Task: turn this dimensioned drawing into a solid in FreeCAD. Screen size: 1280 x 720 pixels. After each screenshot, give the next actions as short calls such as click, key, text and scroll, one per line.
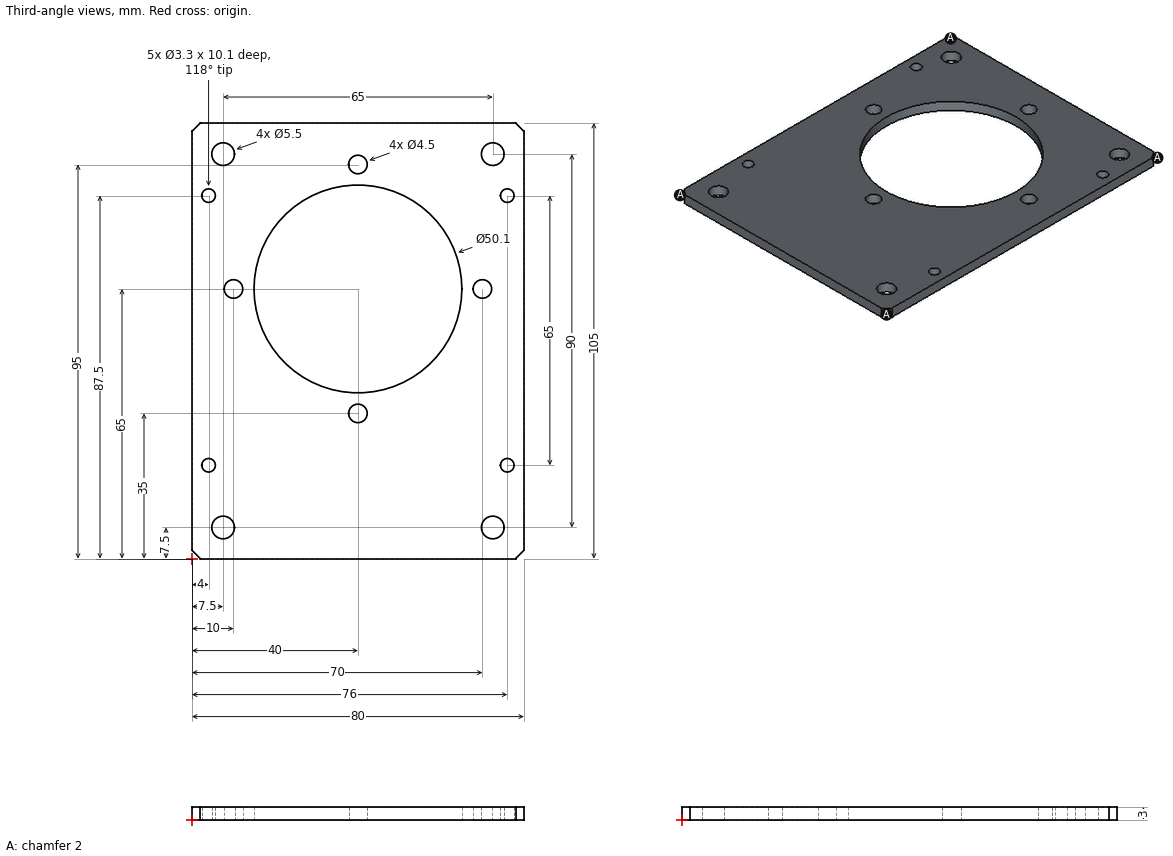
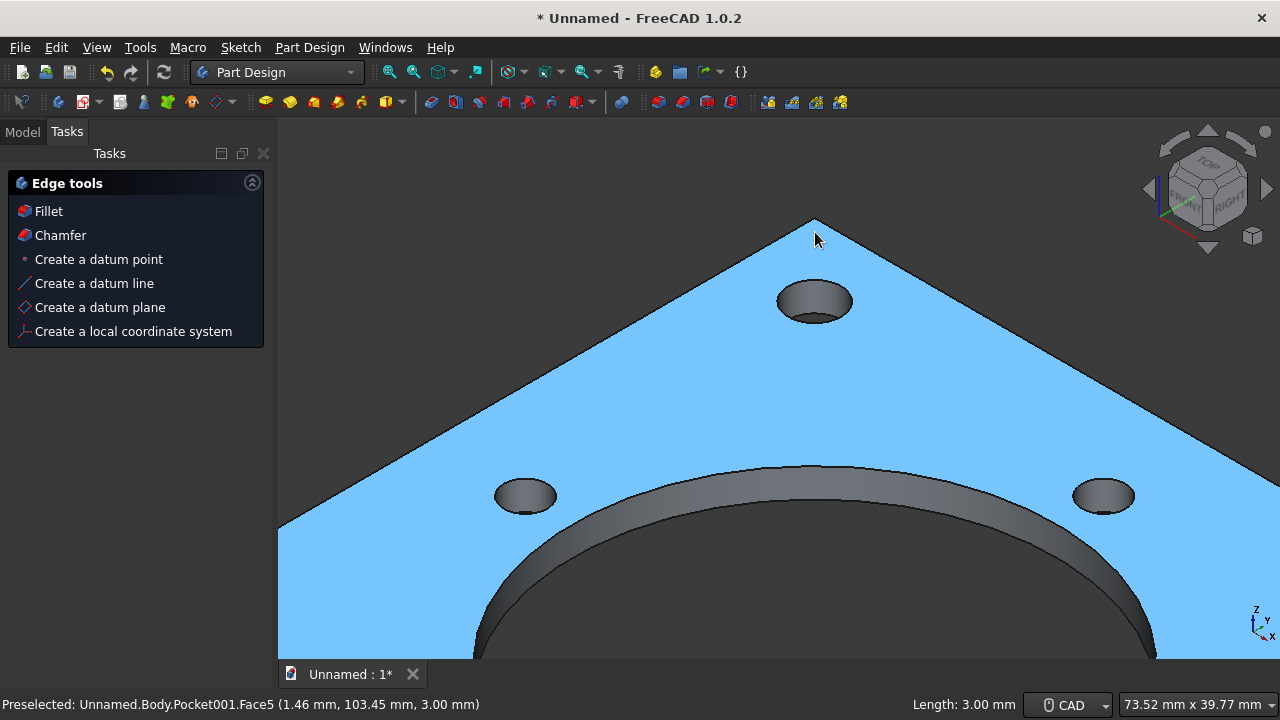
click(390, 72)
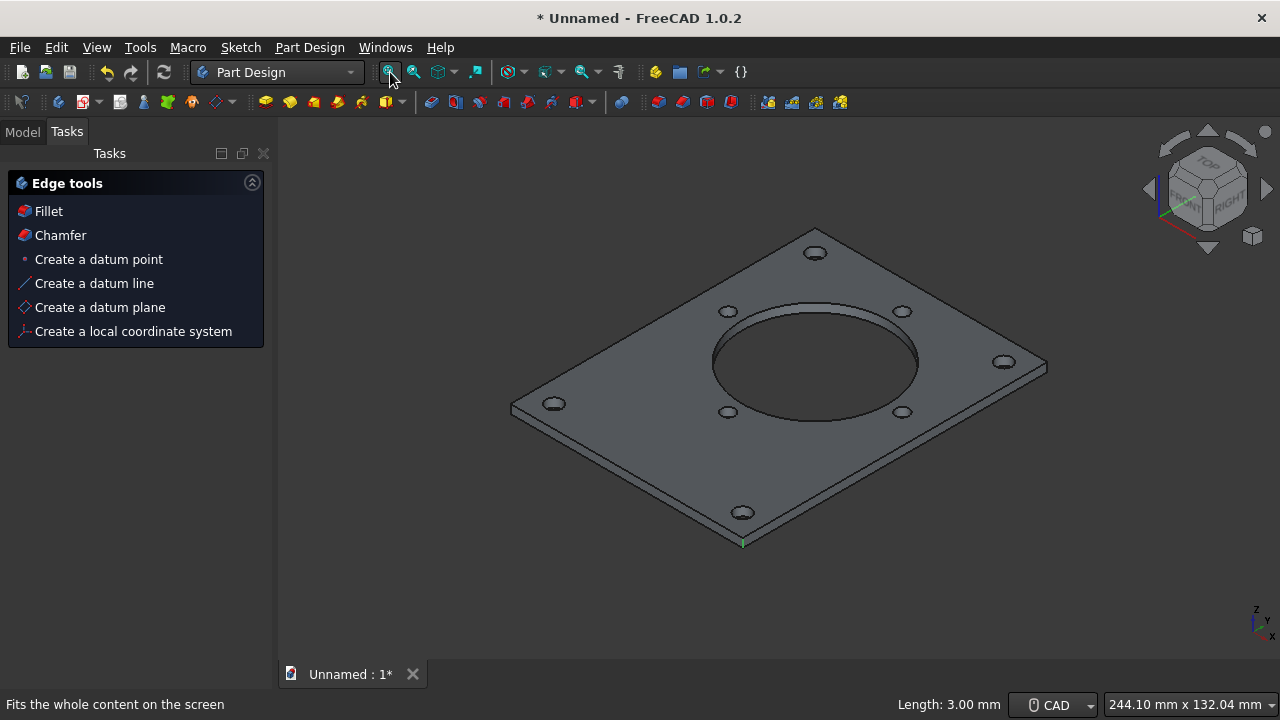
key(2)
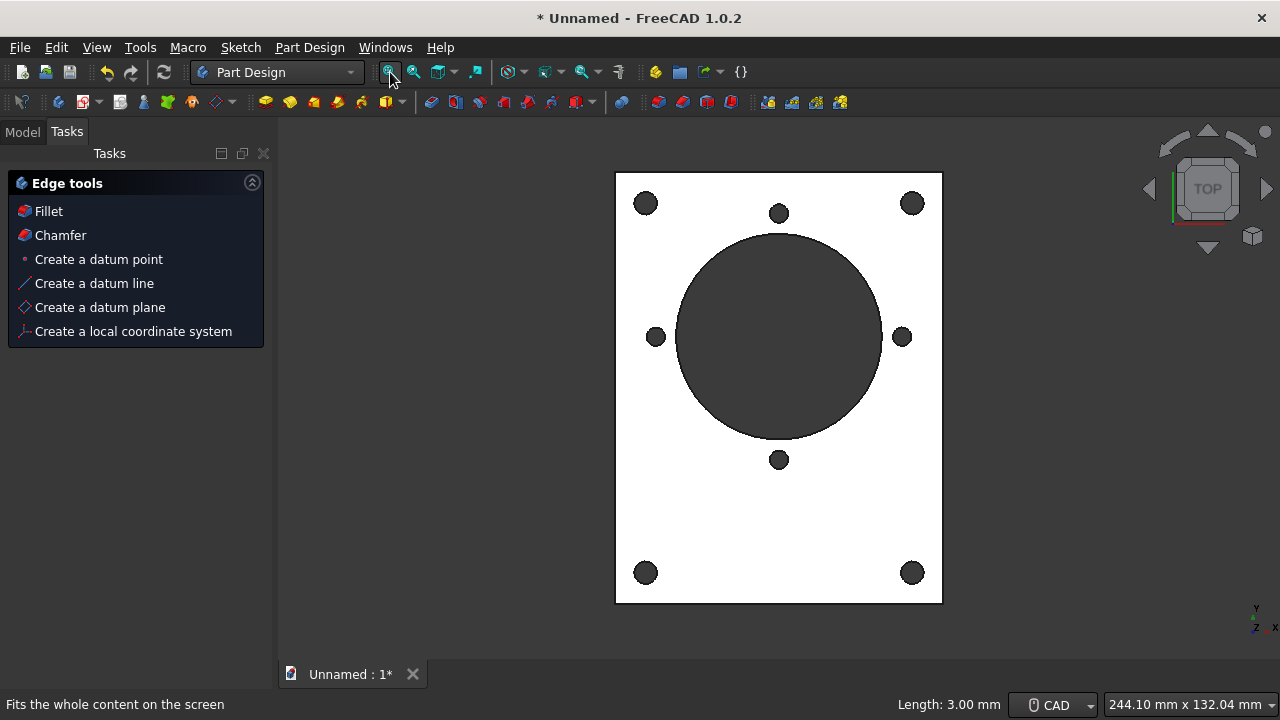
scroll(615, 171, up, 6)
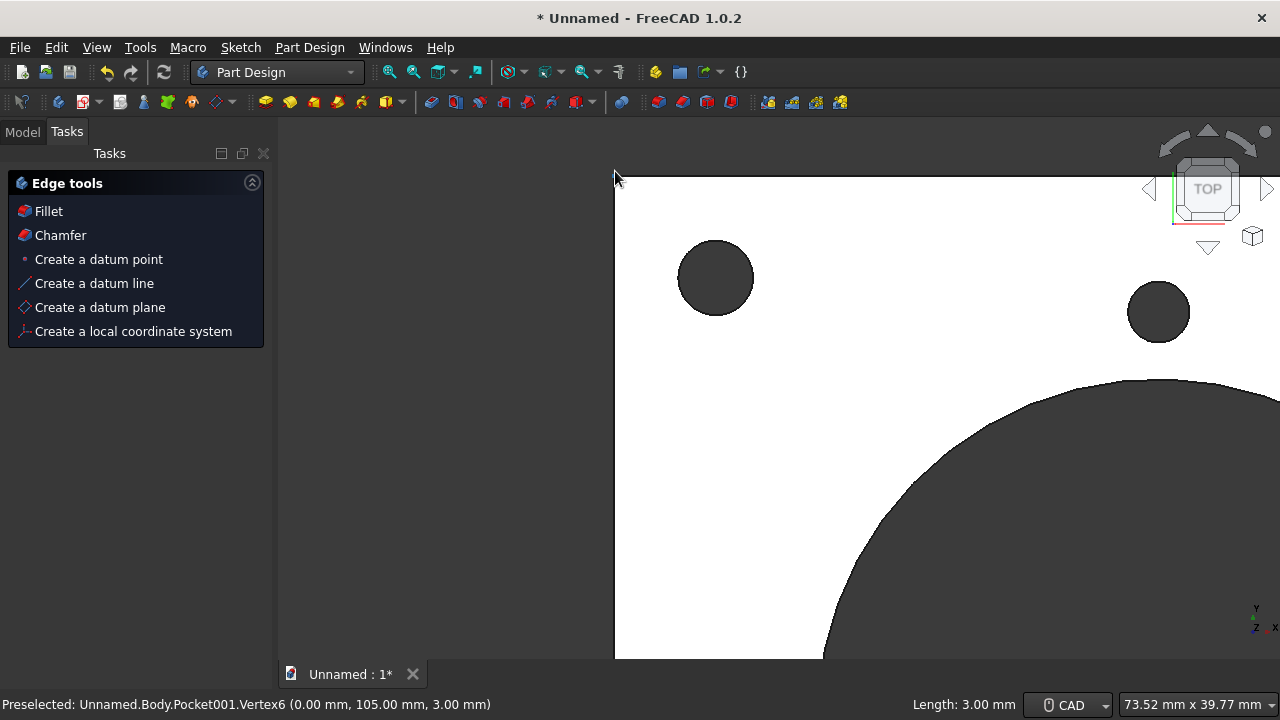
click(390, 72)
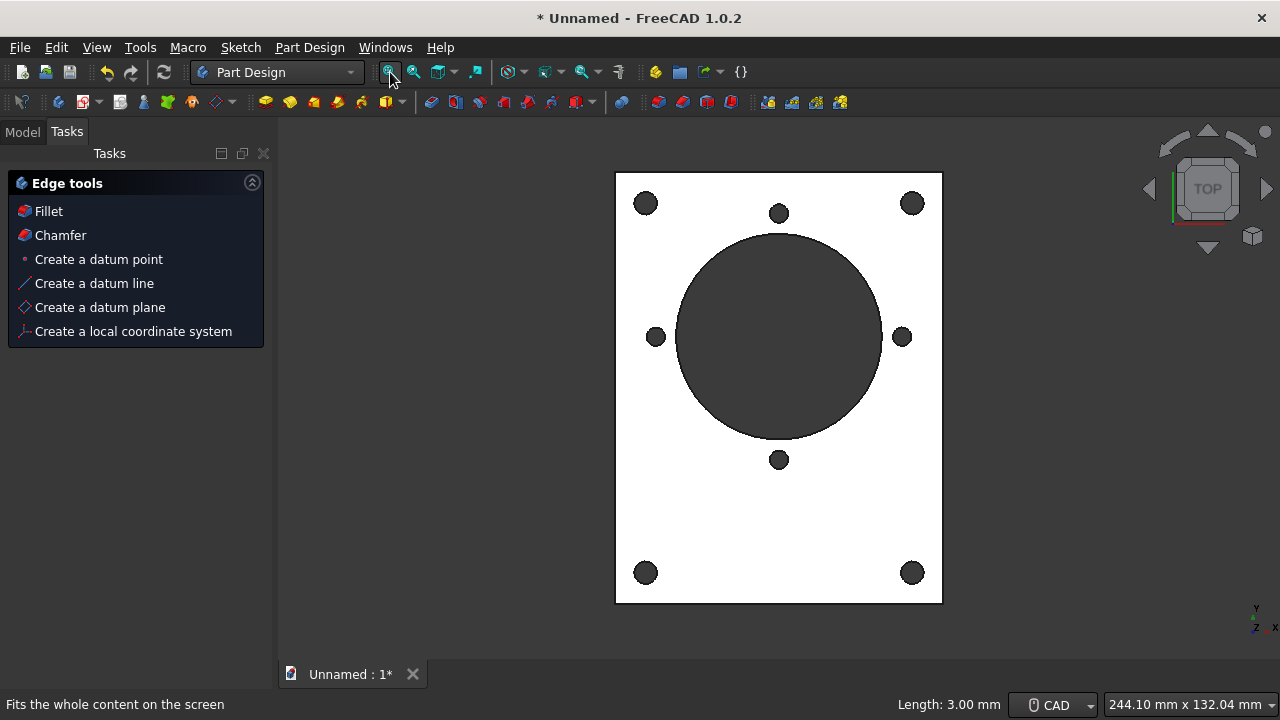
key(1)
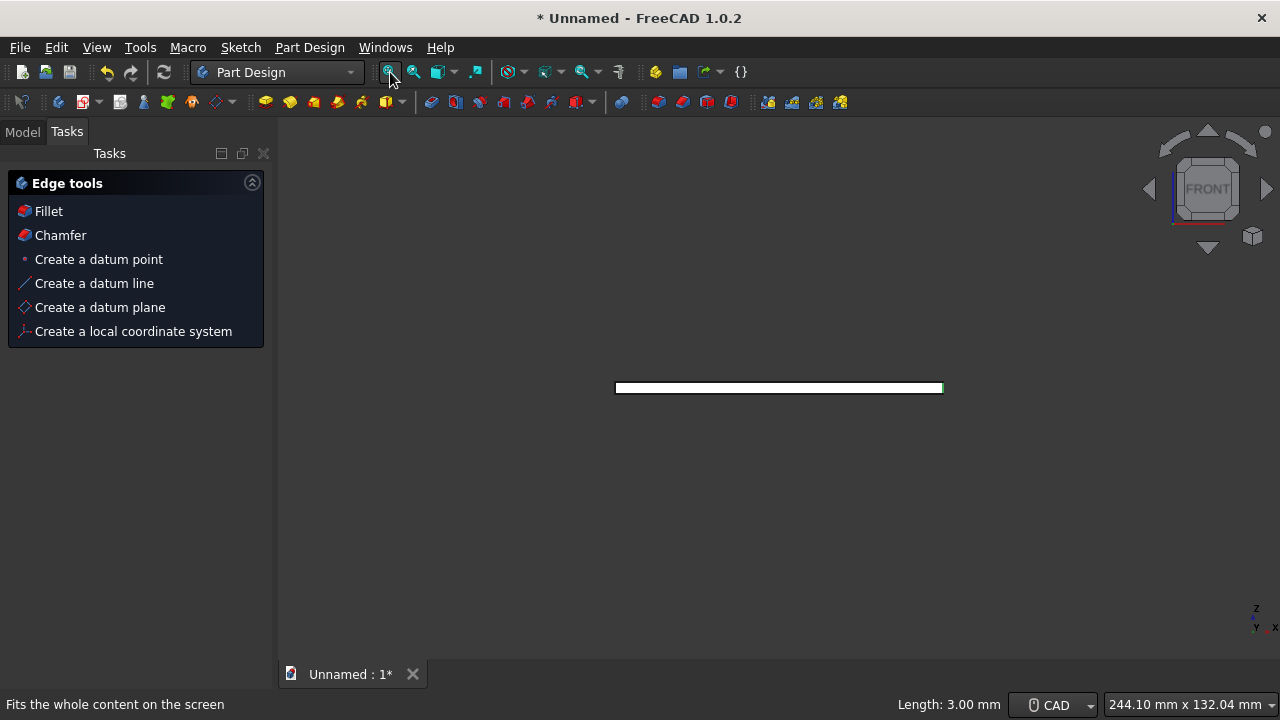
click(390, 72)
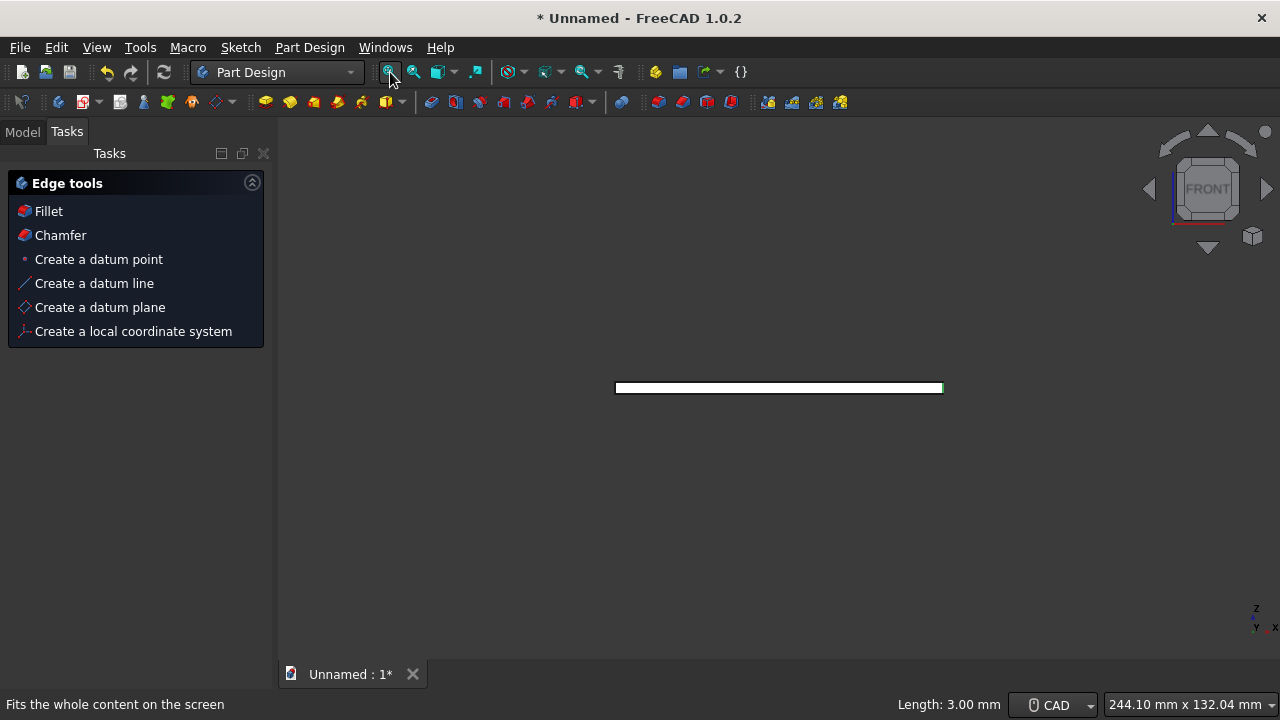
click(615, 387, ctrl)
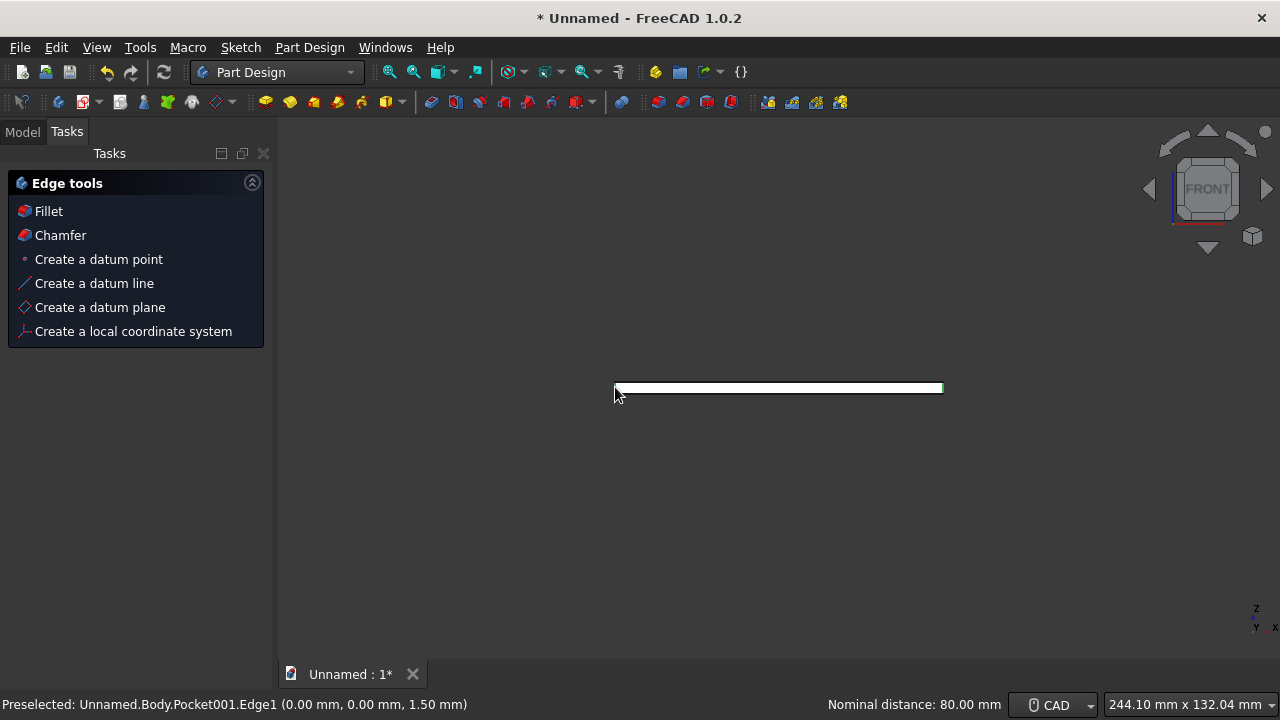
scroll(615, 387, up, 6)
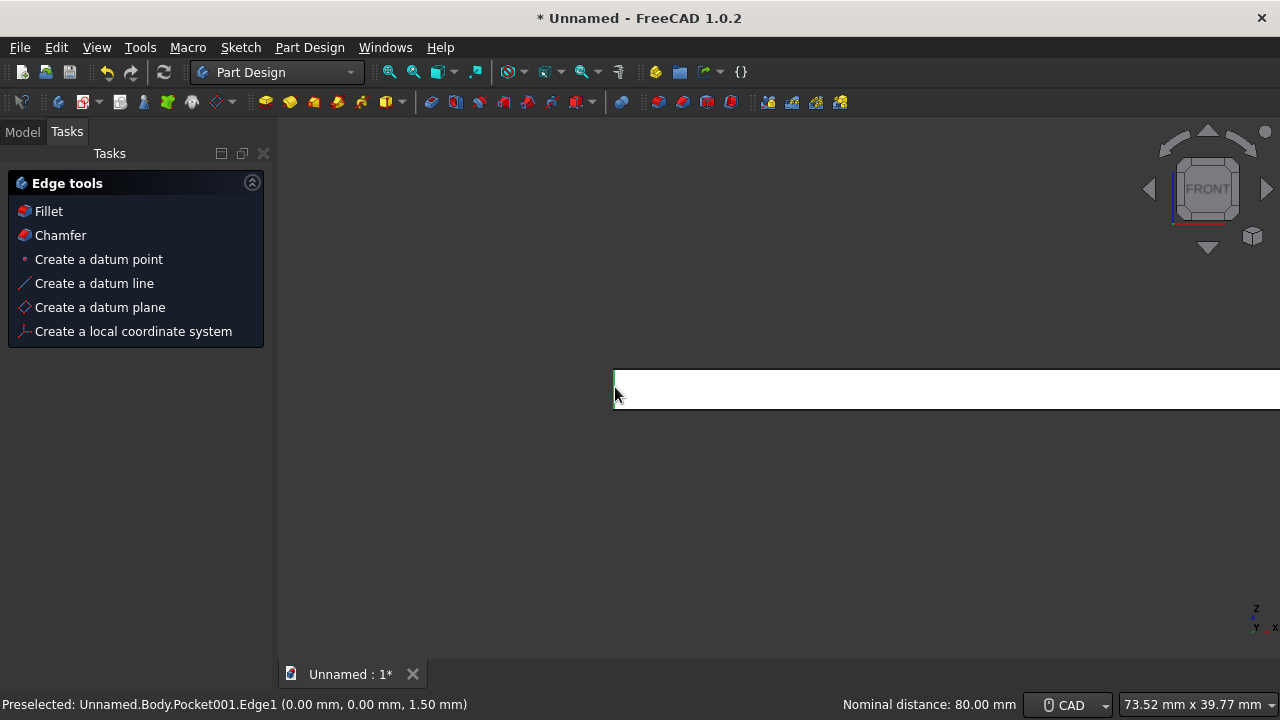
click(390, 72)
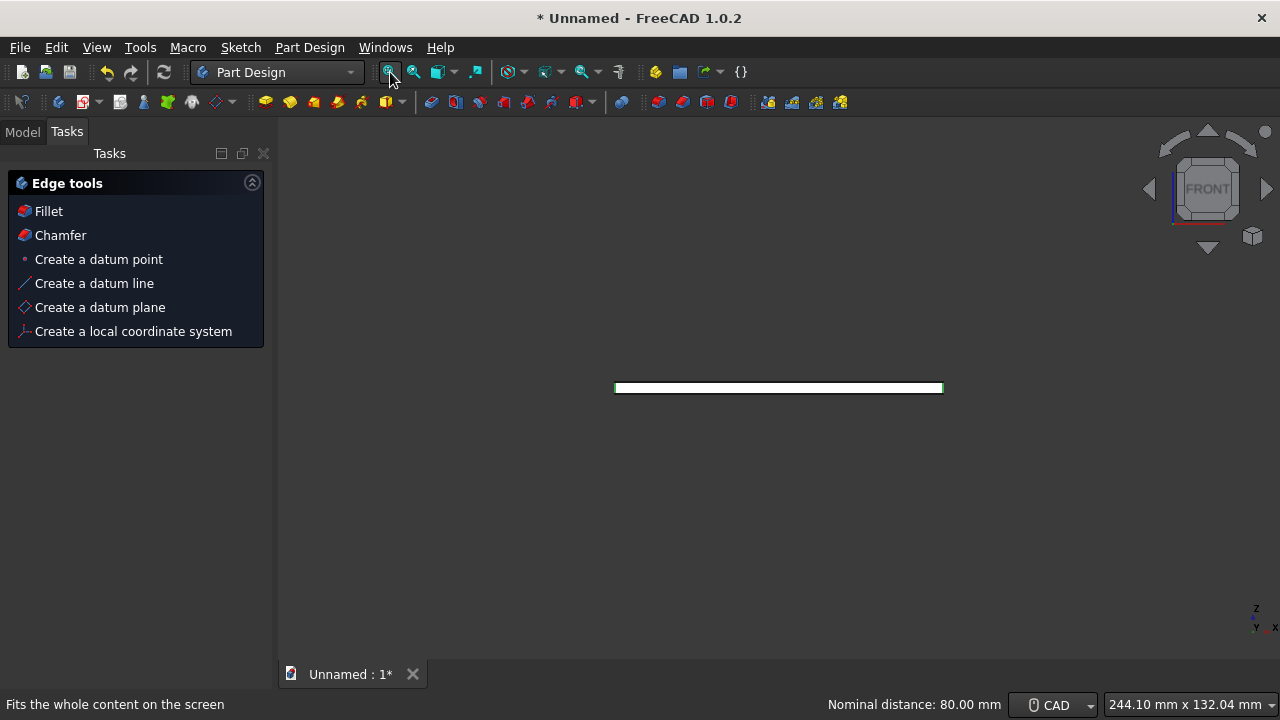
key(3)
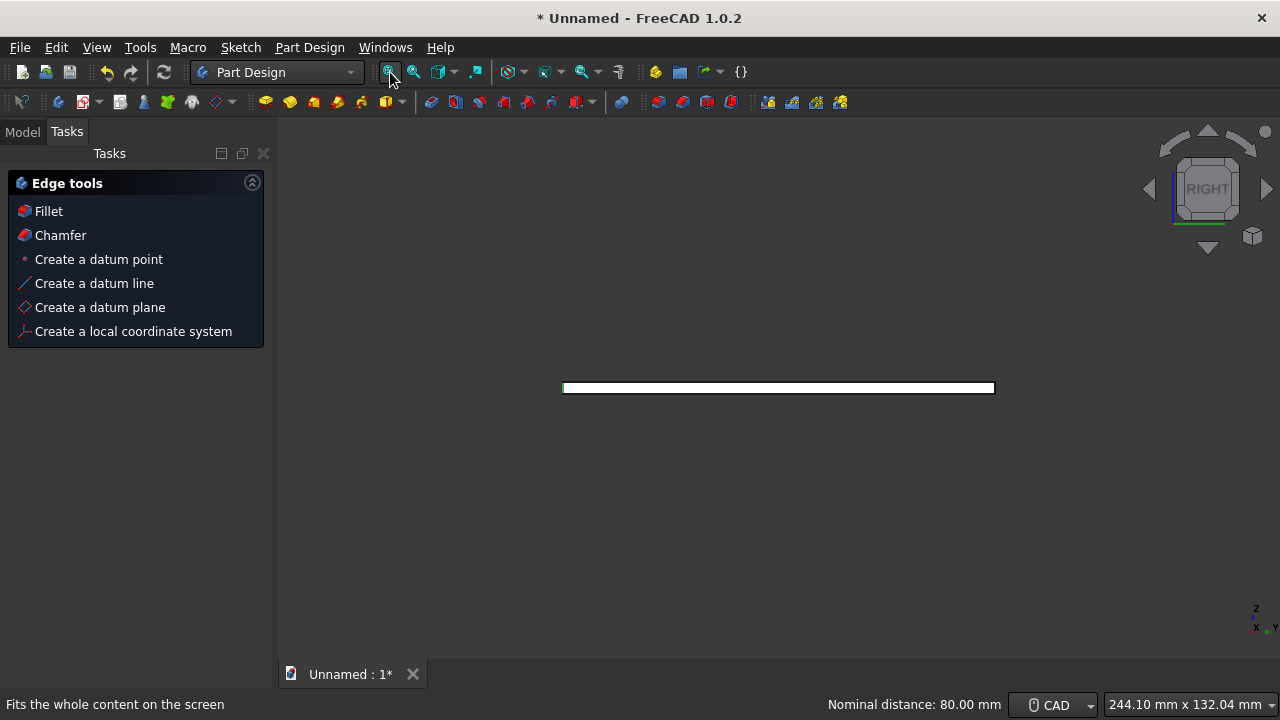
key(v)
key(f)